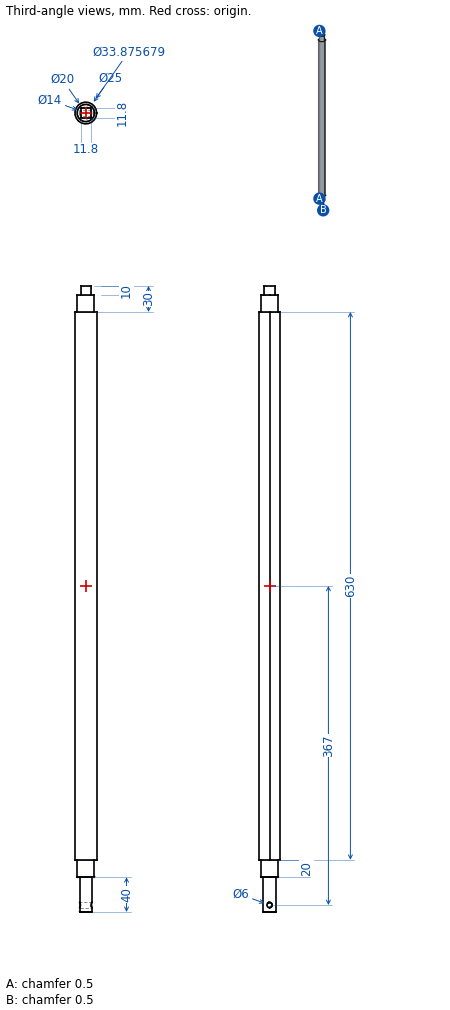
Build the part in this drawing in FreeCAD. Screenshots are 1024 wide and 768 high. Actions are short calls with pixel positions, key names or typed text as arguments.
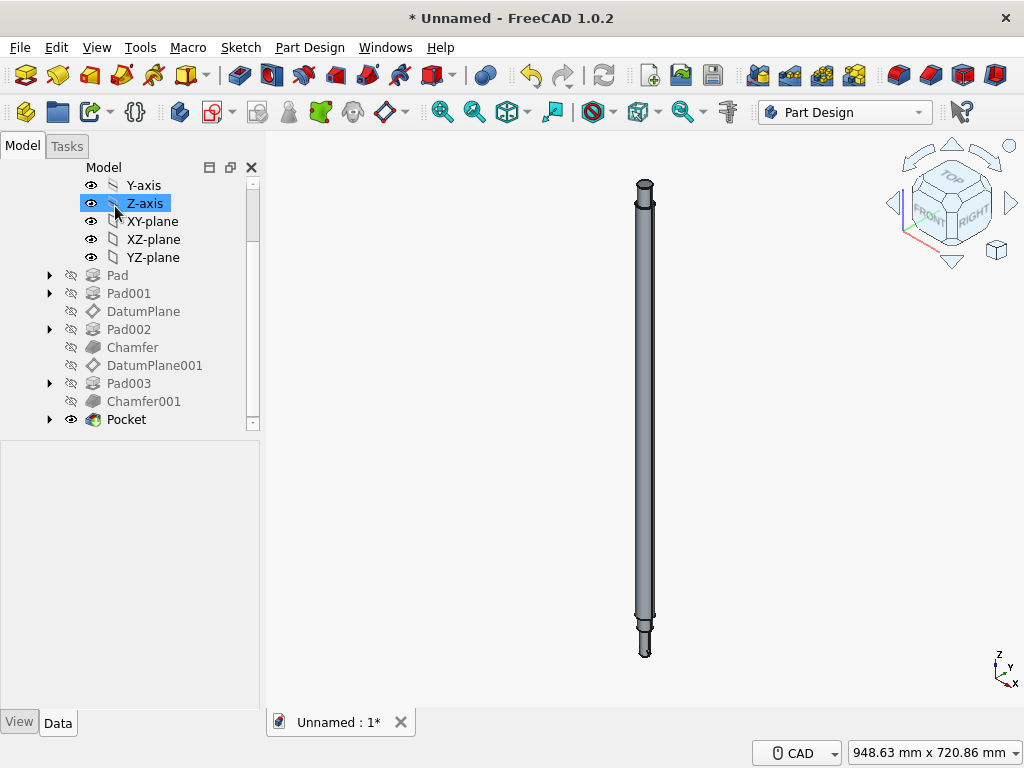
key(2)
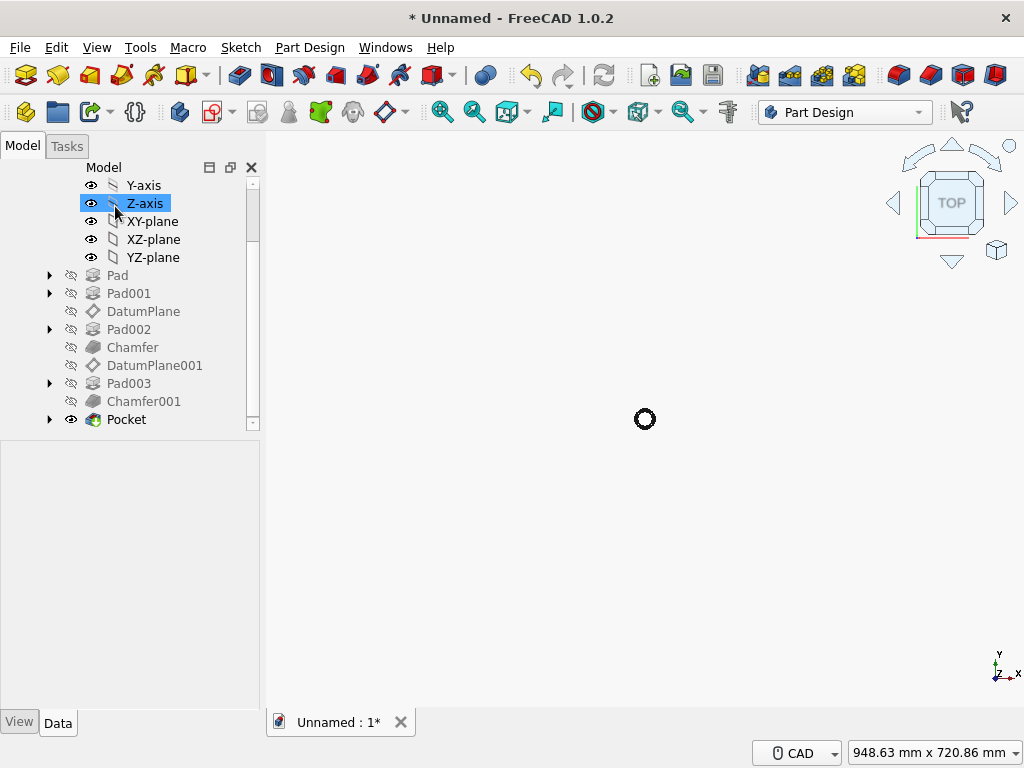
click(444, 112)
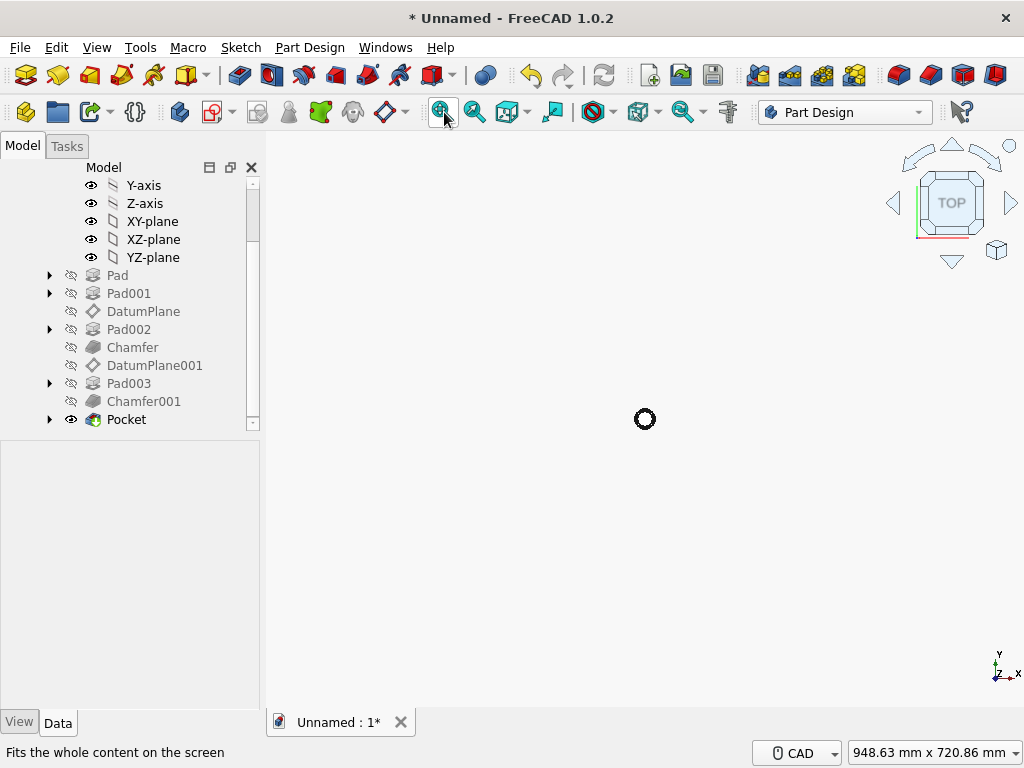
key(0)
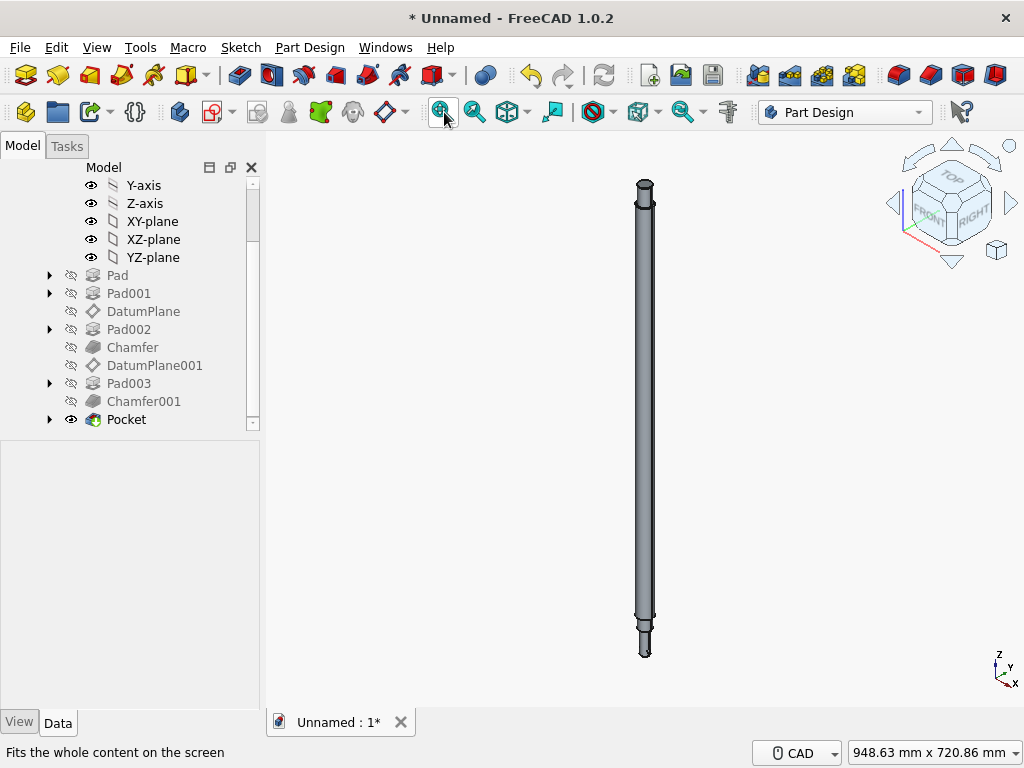
key(1)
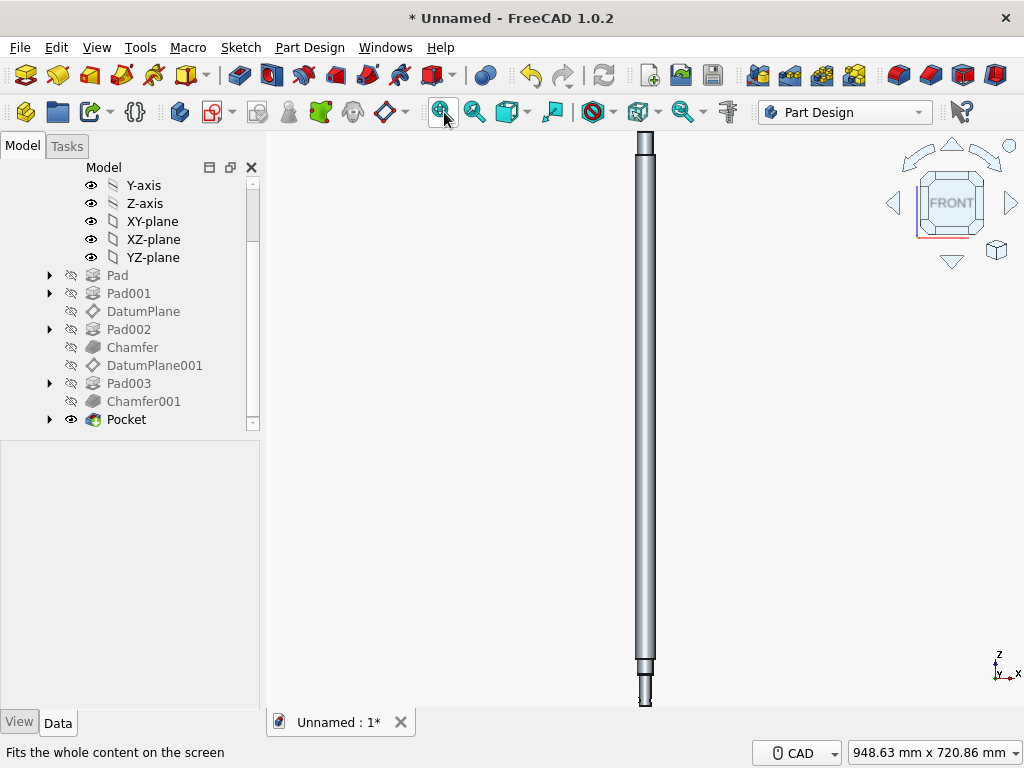
click(444, 112)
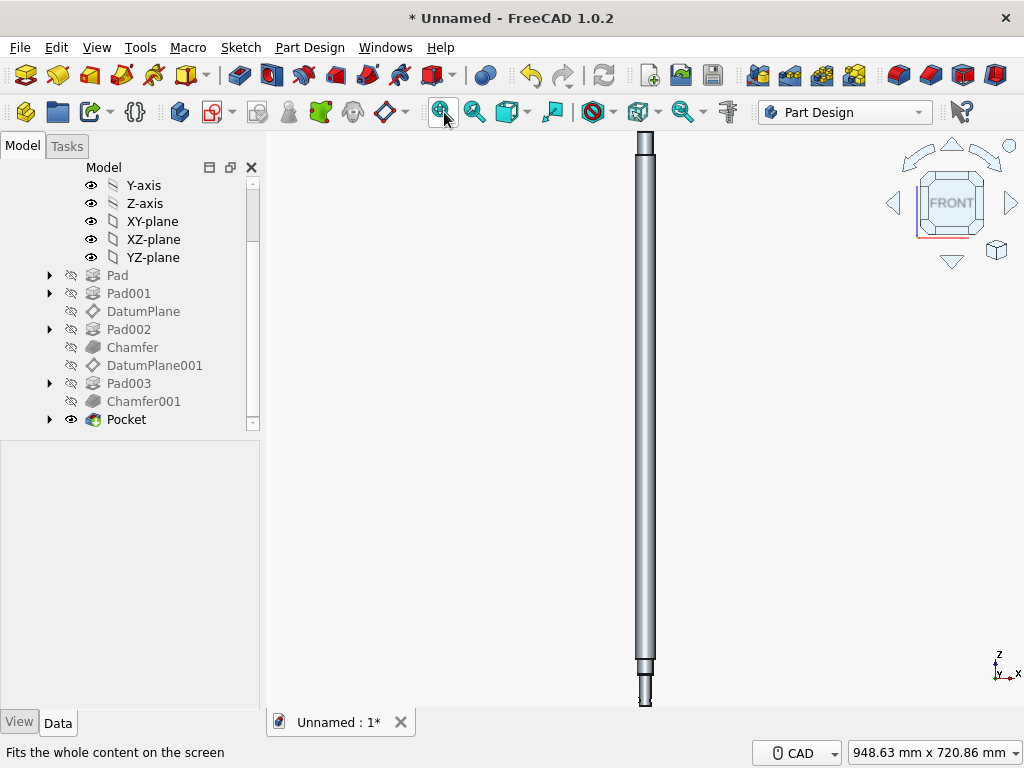
scroll(160, 307, down, 3)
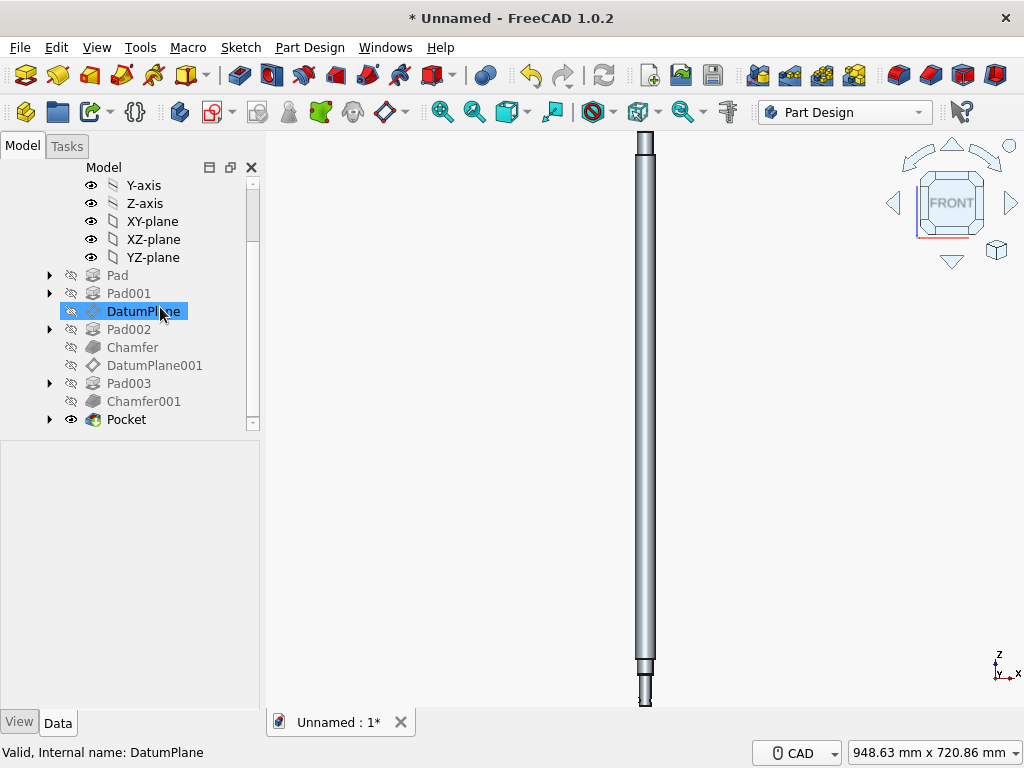
scroll(160, 307, up, 15)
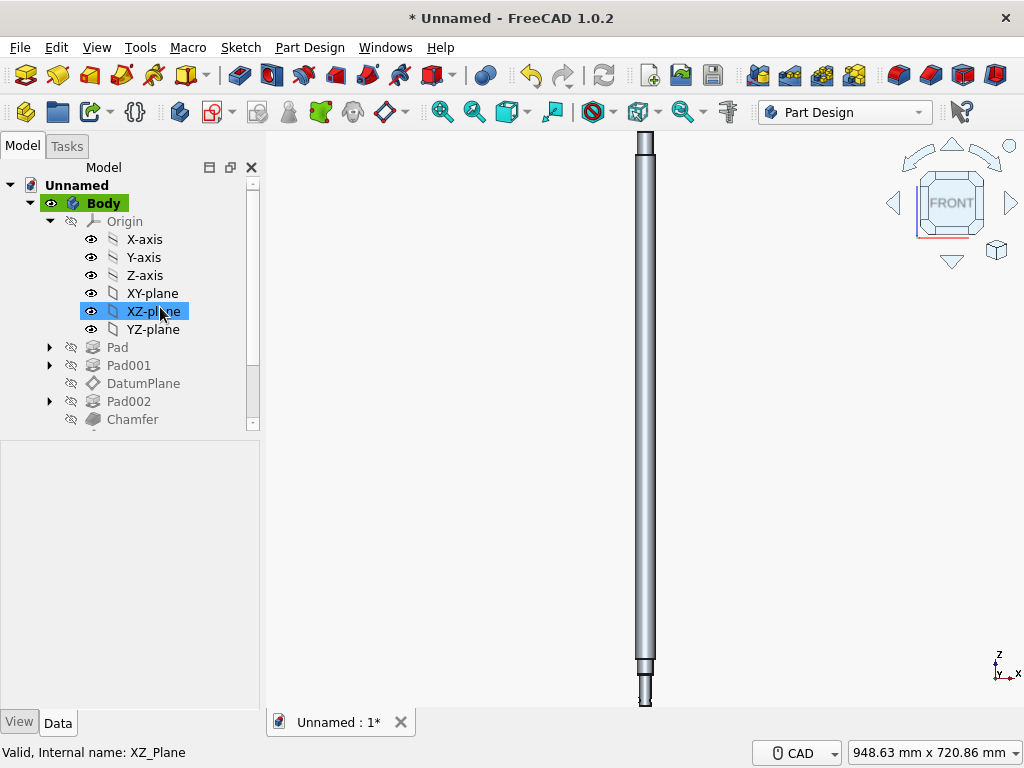
click(136, 293)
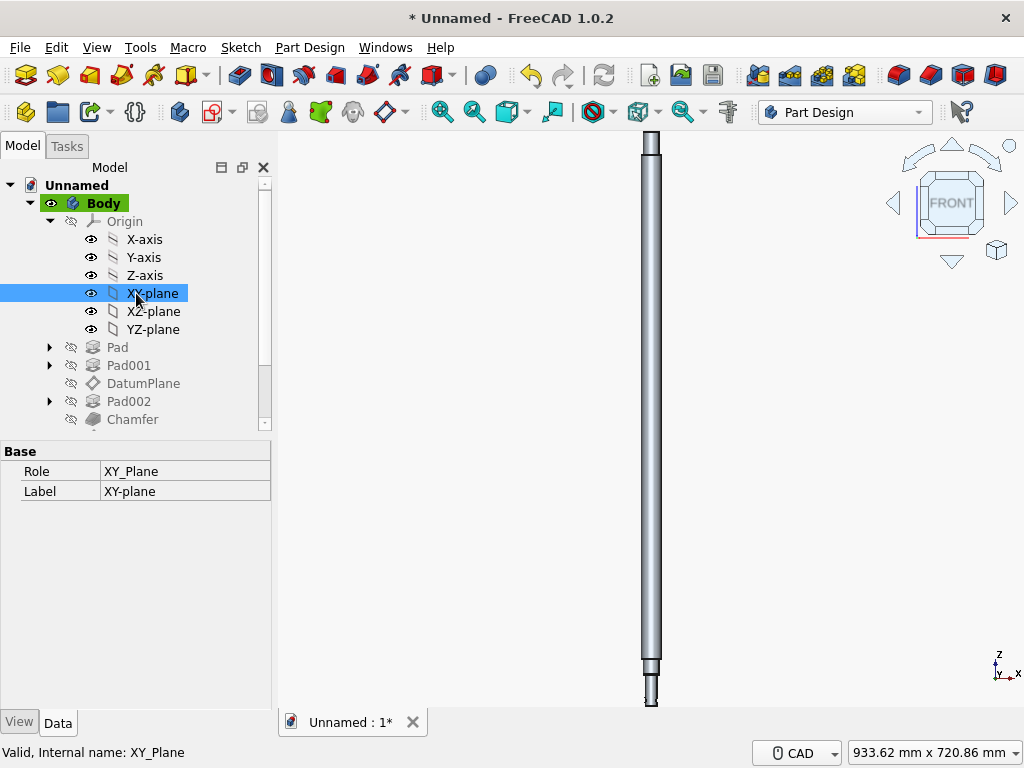
click(386, 112)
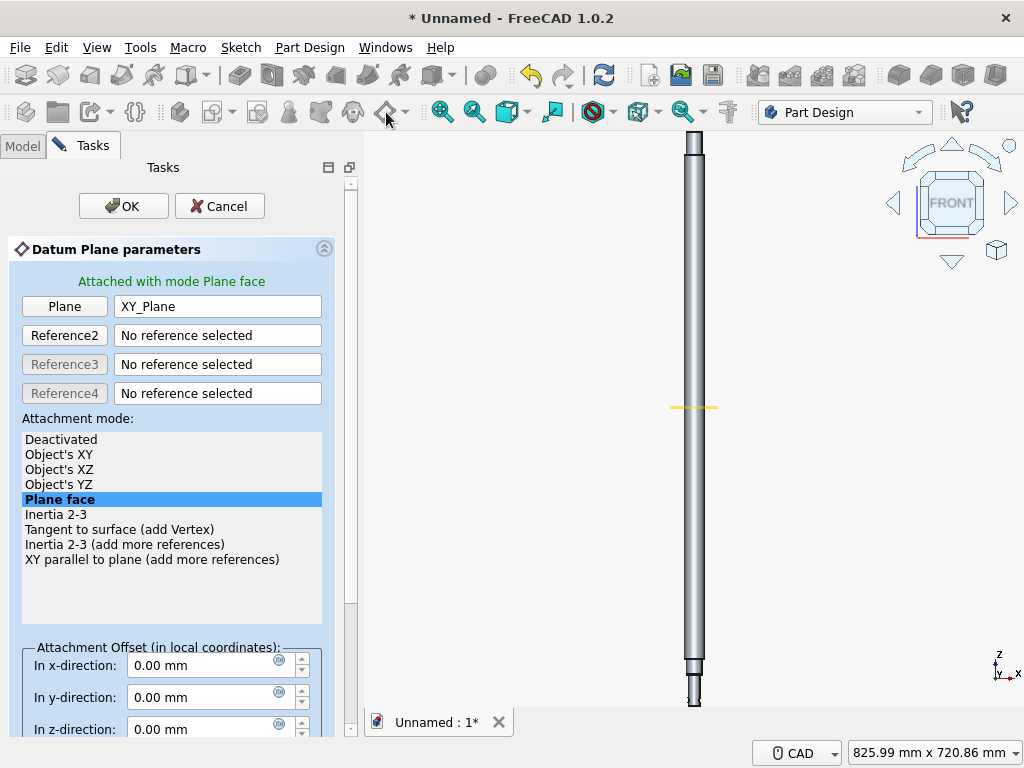
scroll(351, 456, down, 2)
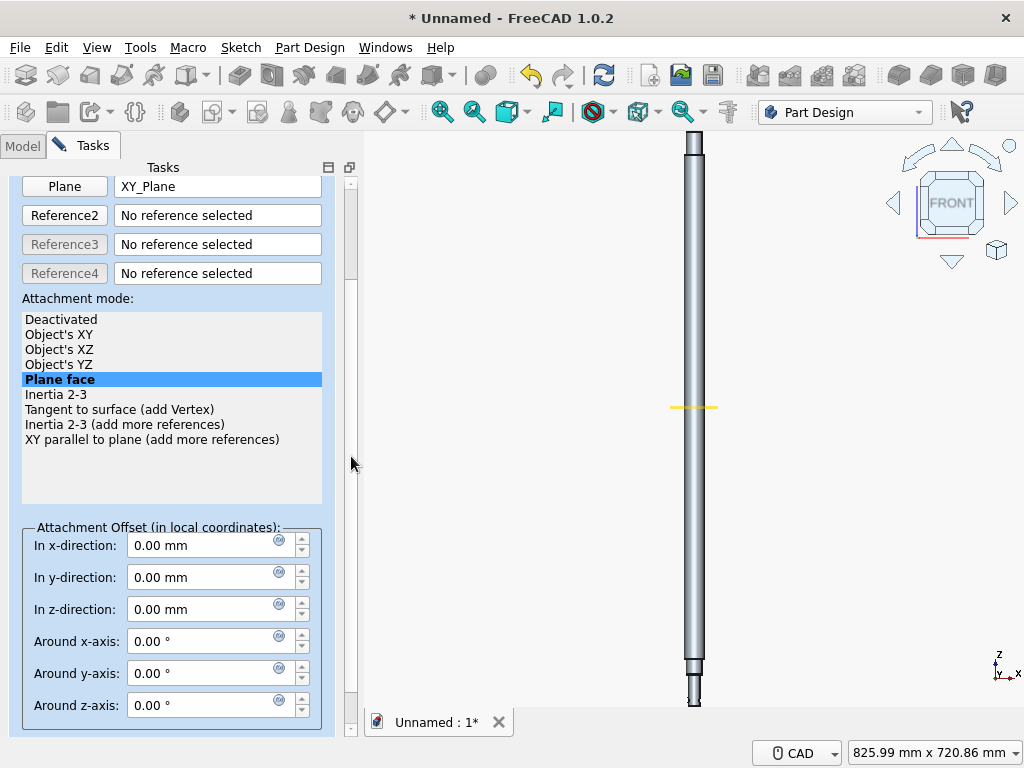
triple_click(210, 609)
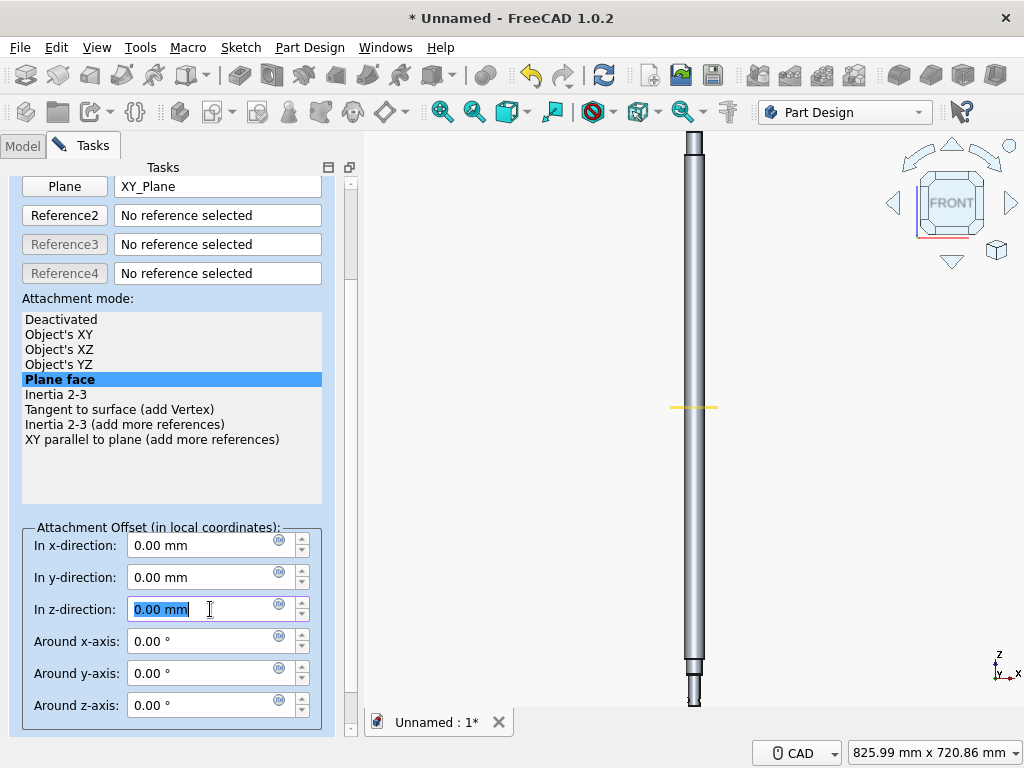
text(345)
key(Tab)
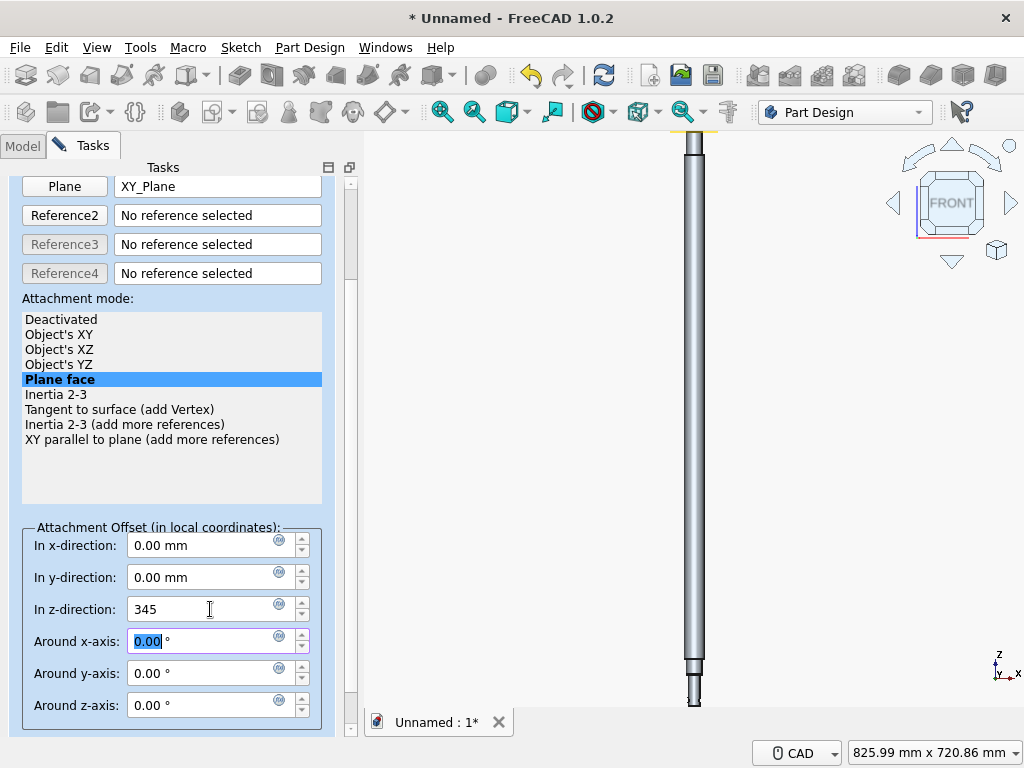
scroll(351, 456, up, 3)